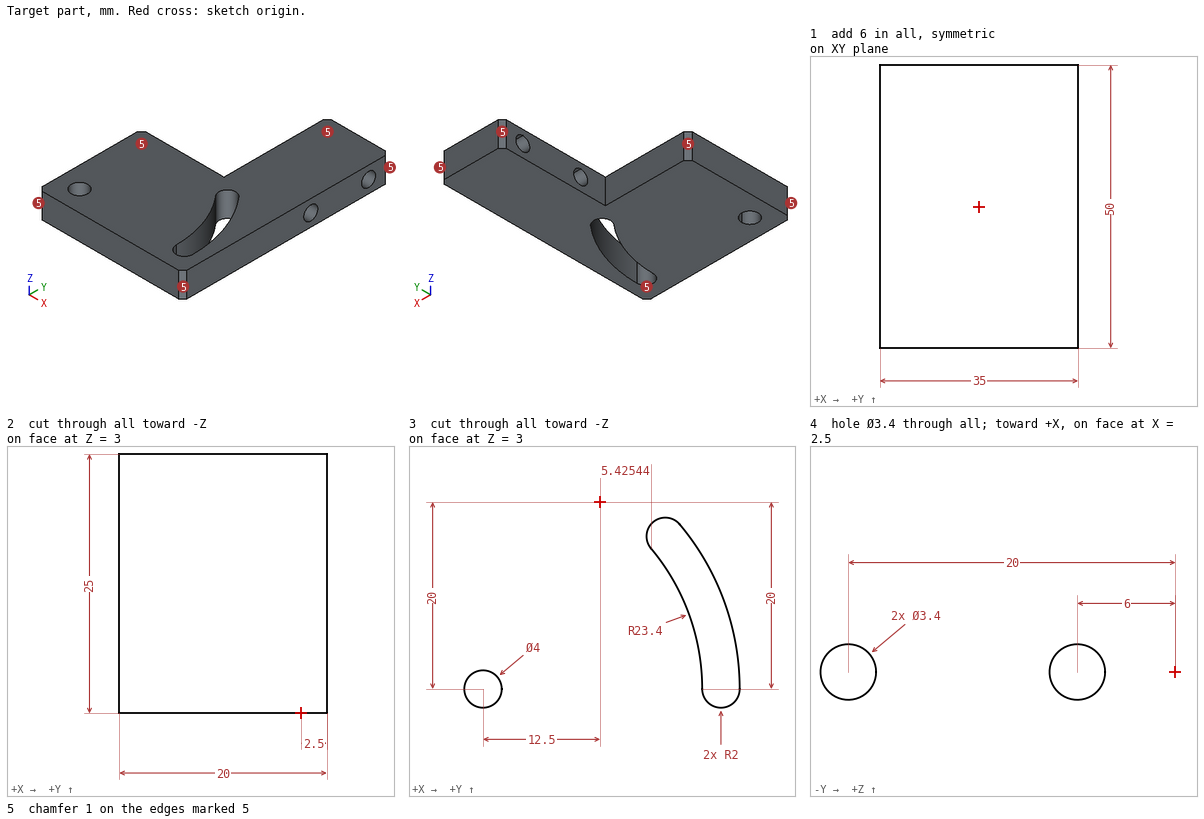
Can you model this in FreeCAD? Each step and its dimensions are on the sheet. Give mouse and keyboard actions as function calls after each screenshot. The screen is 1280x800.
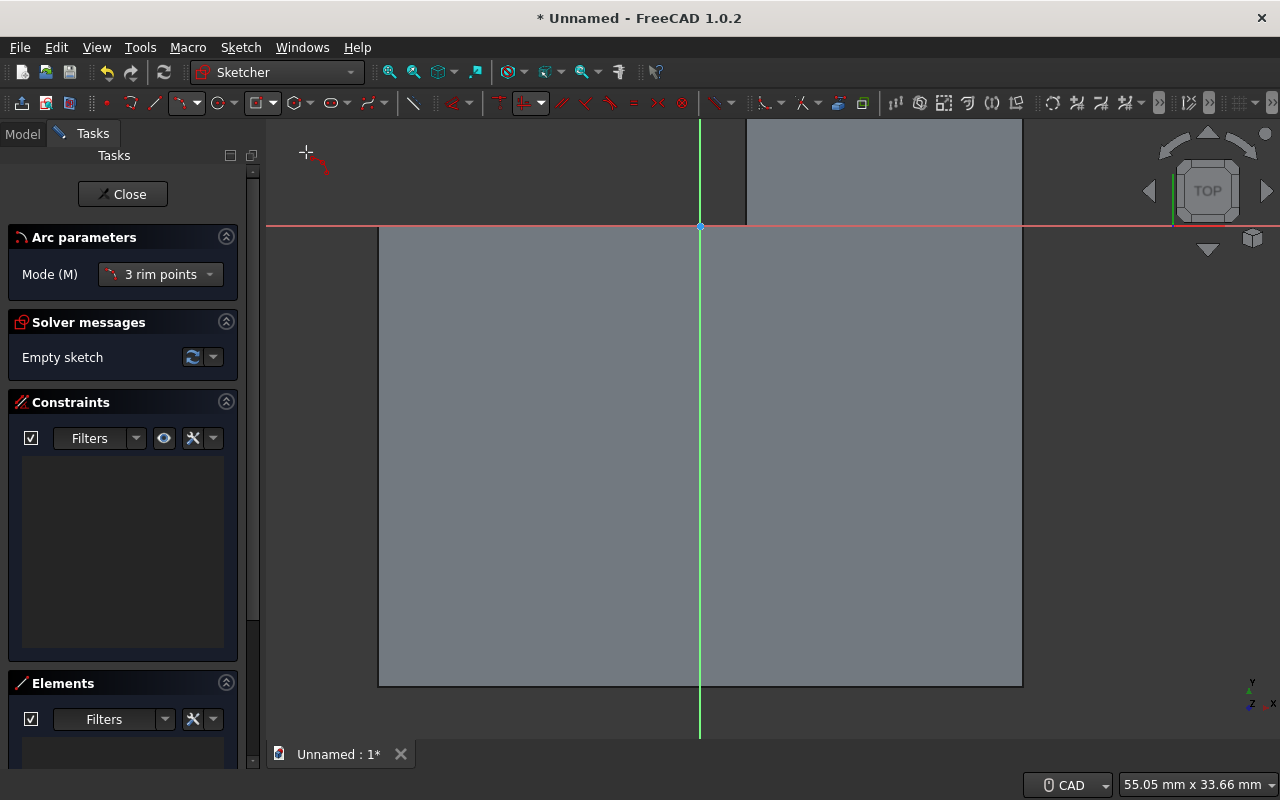
click(800, 317)
click(901, 594)
click(875, 447)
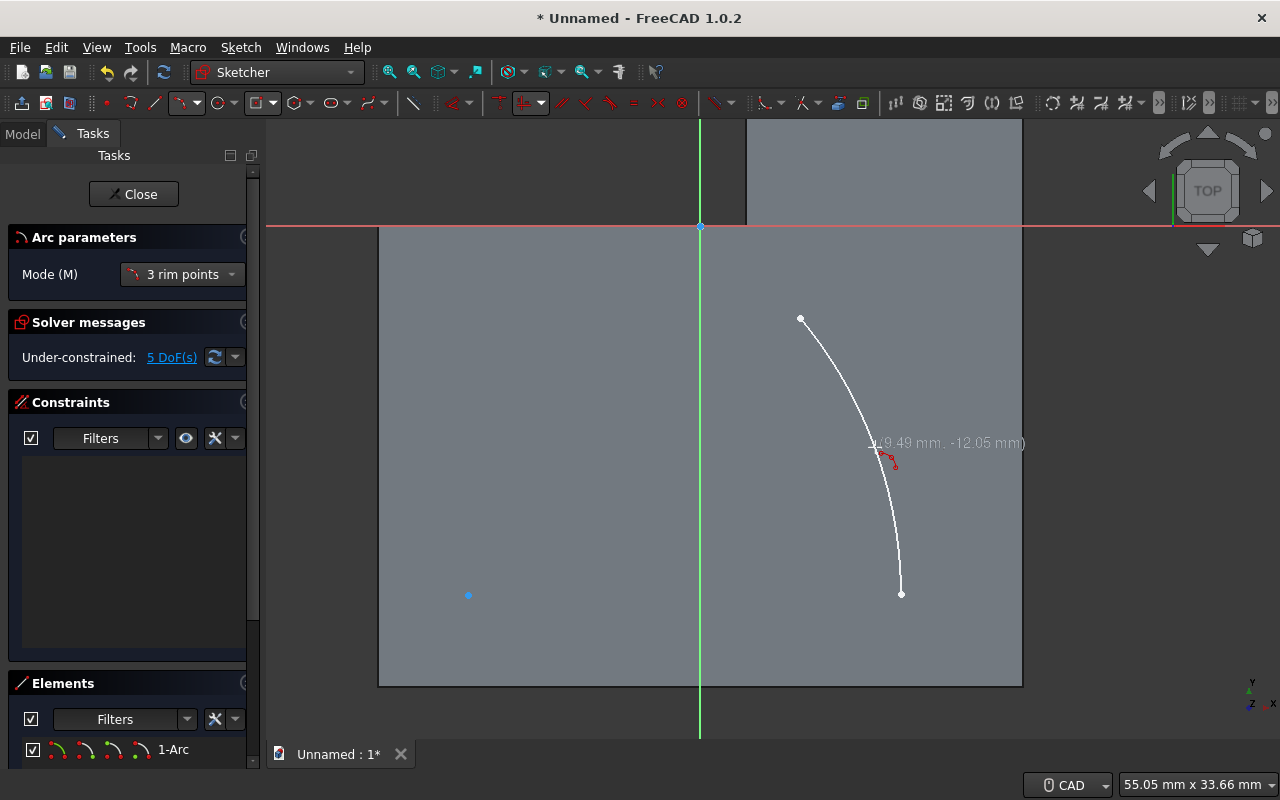
click(901, 595)
click(975, 594)
click(938, 631)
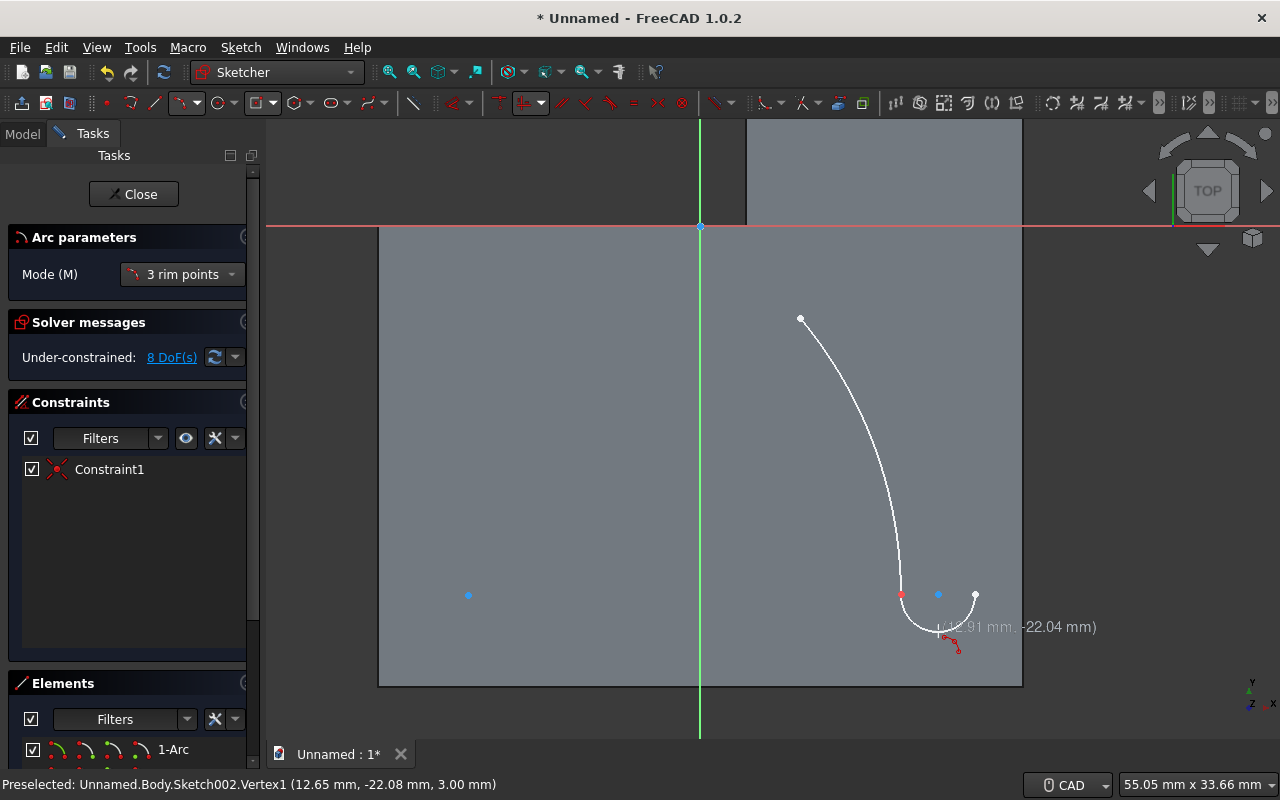
click(975, 595)
click(857, 270)
click(944, 422)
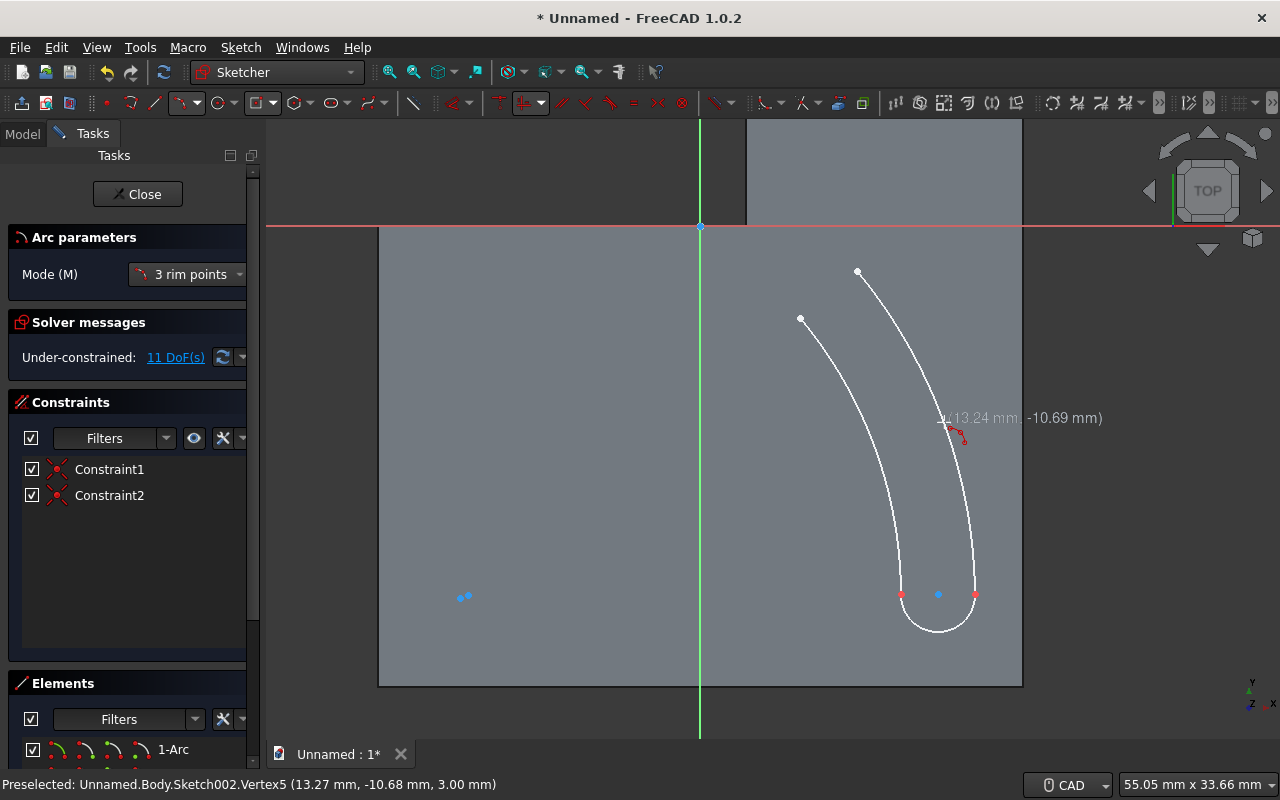
click(857, 271)
click(800, 318)
click(805, 265)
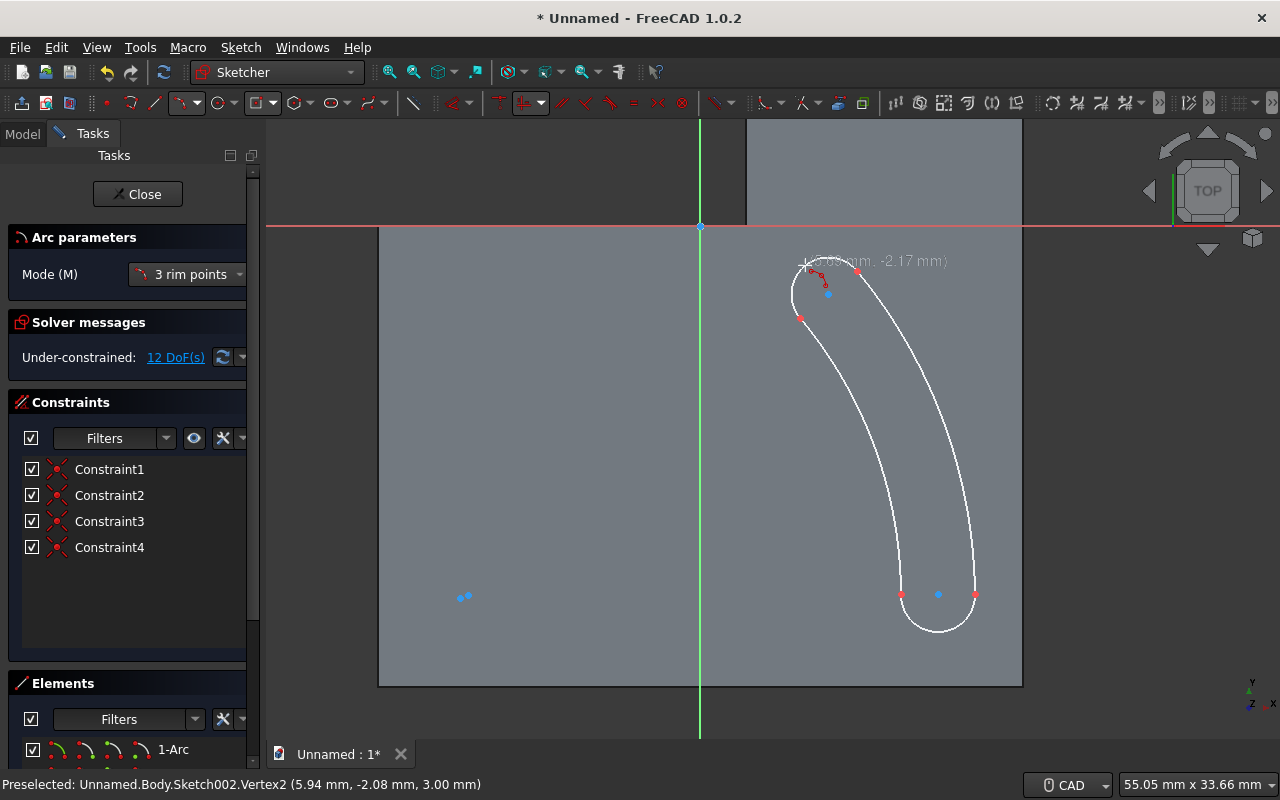
click(218, 104)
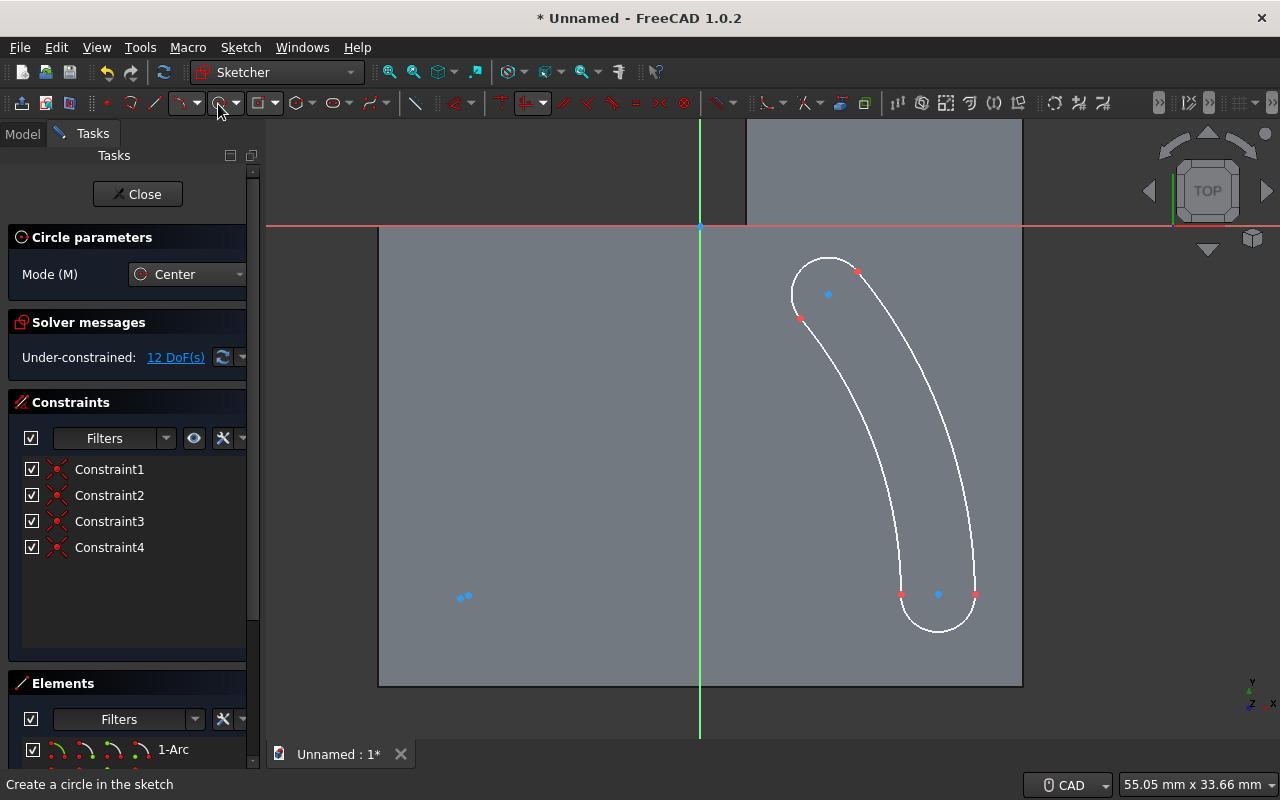
click(470, 594)
click(496, 568)
key(Escape)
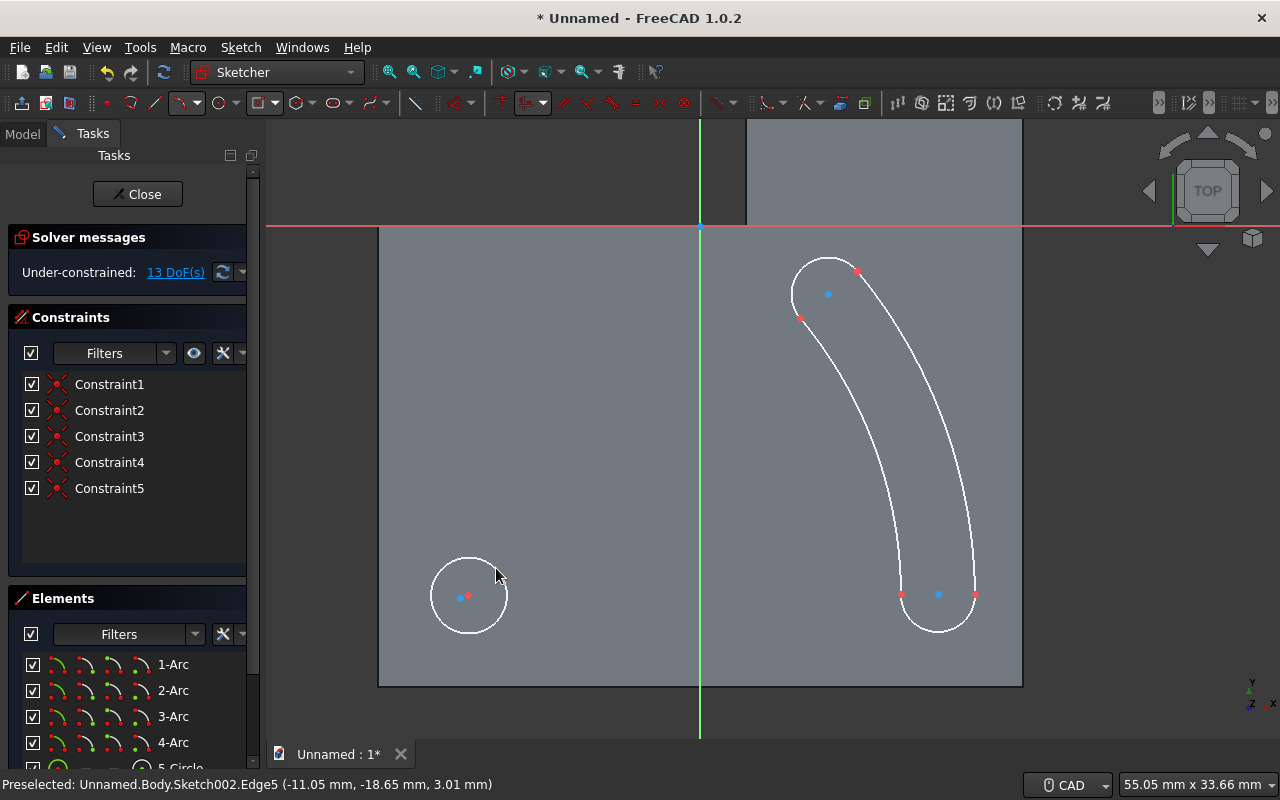
click(891, 505)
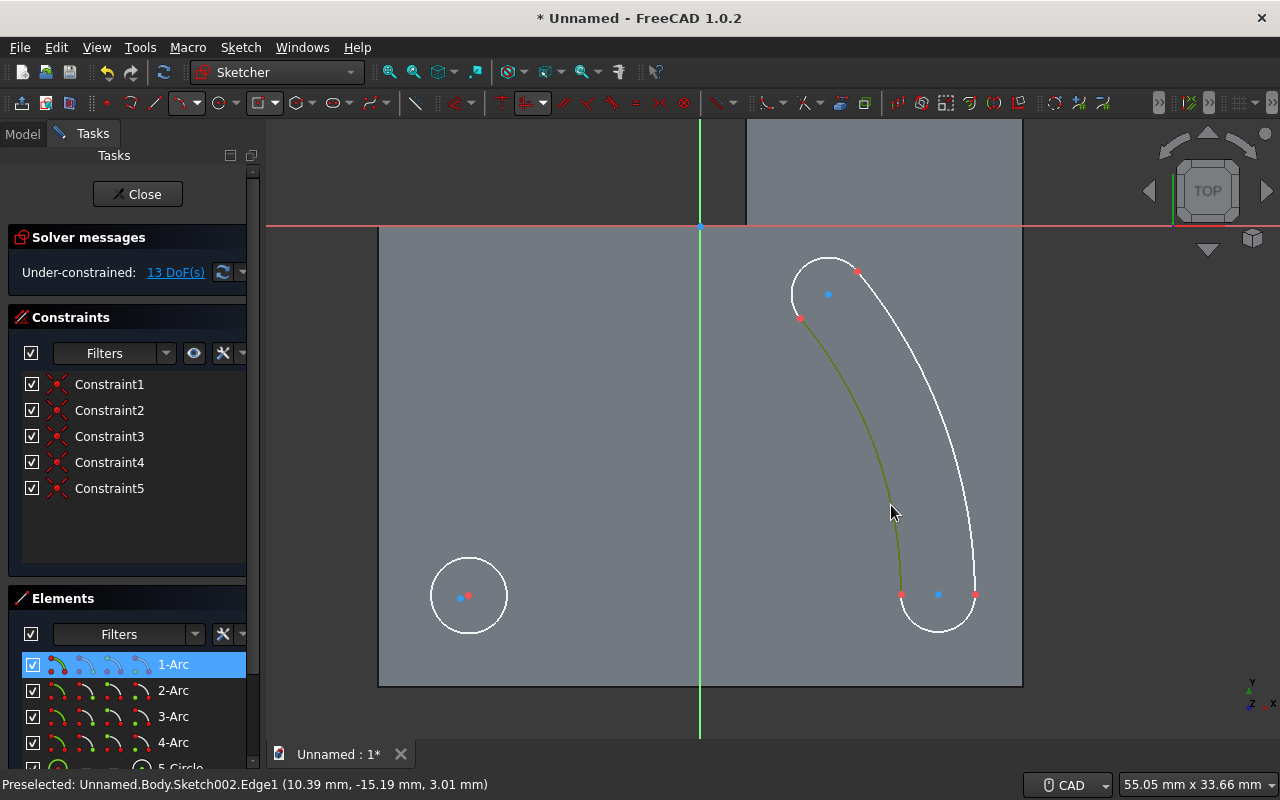
click(916, 625)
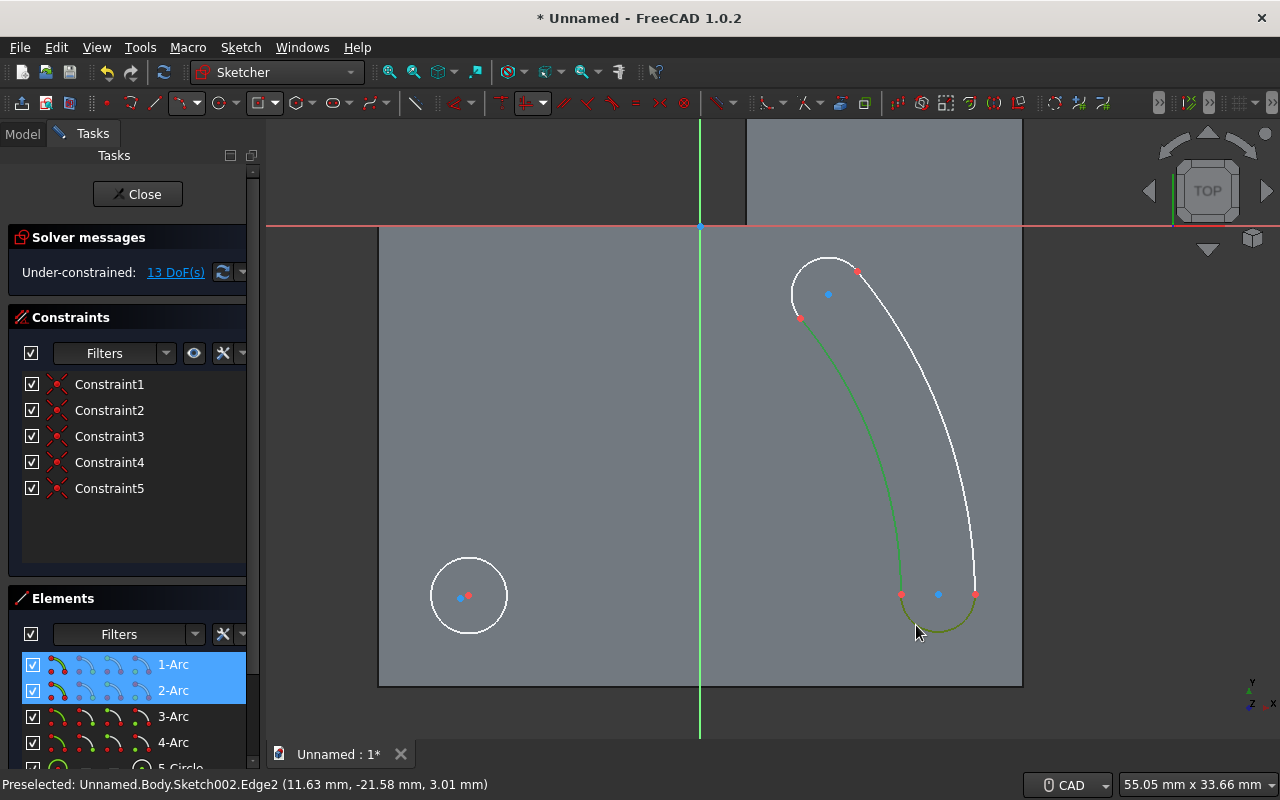
click(612, 104)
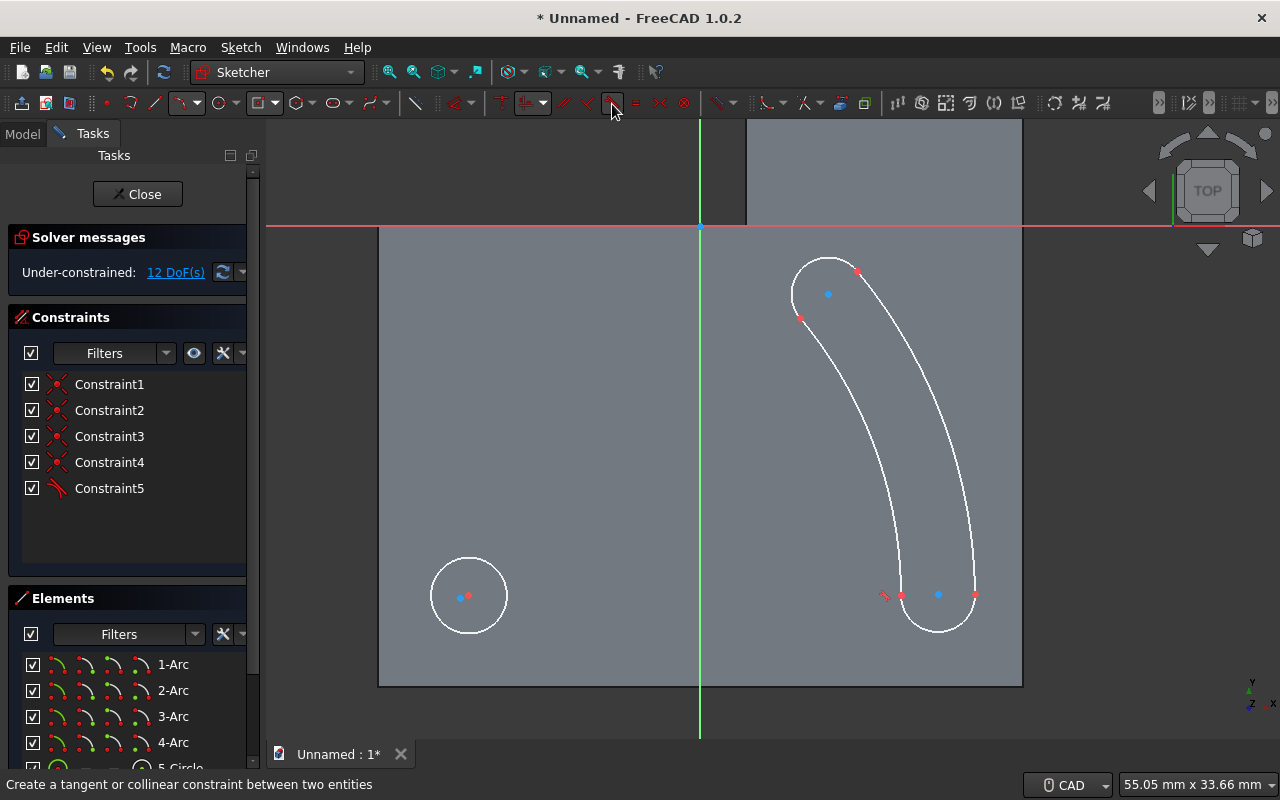
click(891, 505)